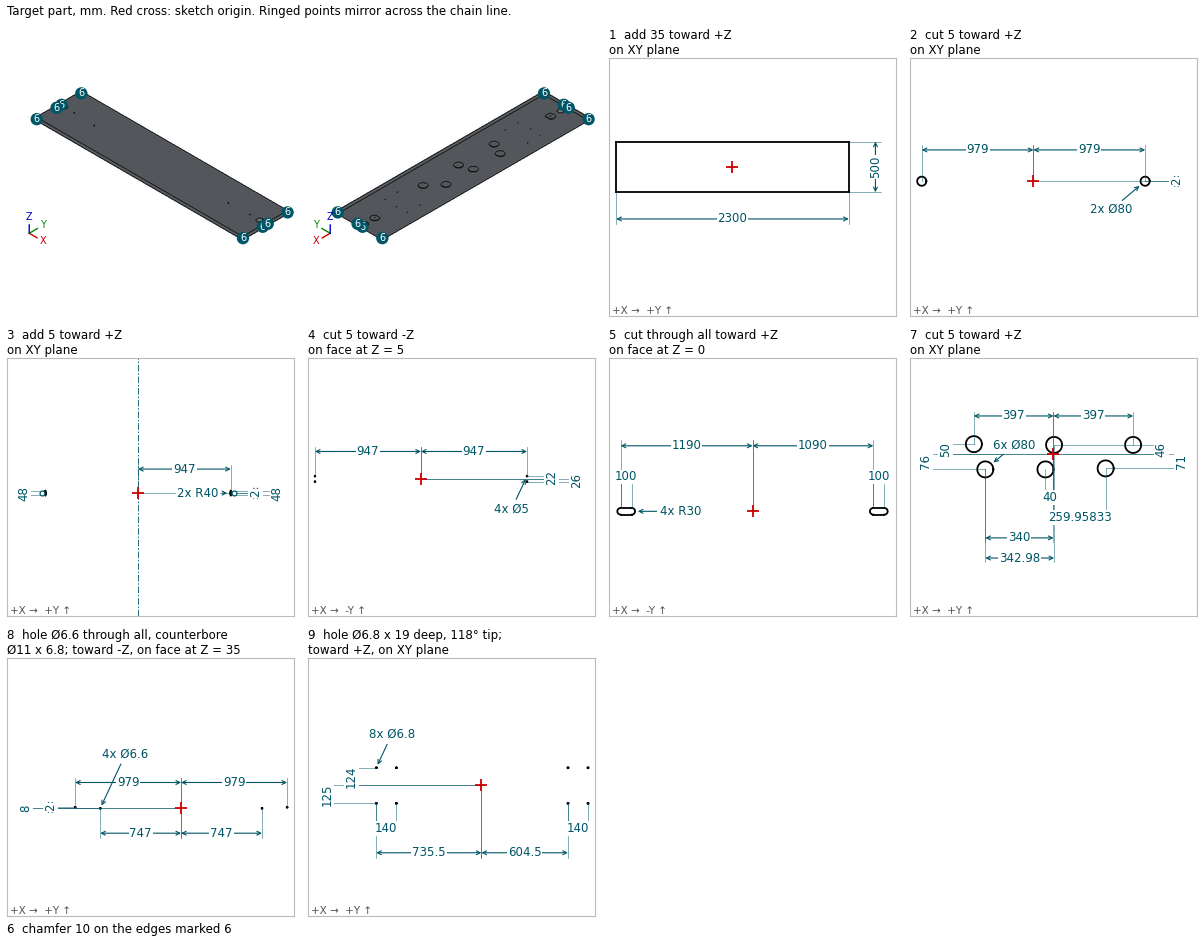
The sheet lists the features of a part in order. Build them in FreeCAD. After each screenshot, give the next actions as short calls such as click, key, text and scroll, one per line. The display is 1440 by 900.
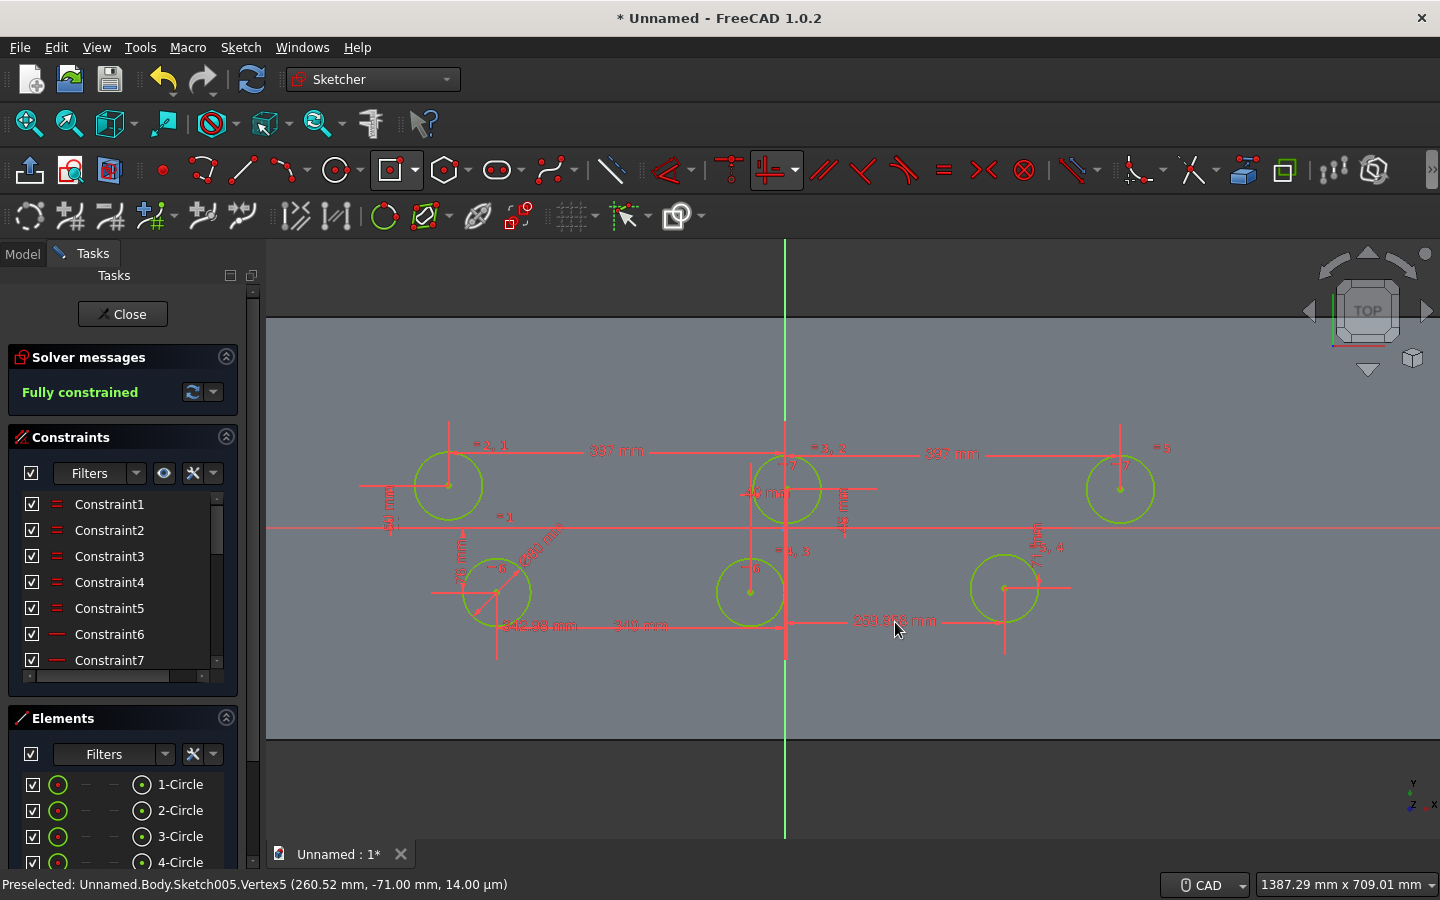
click(123, 314)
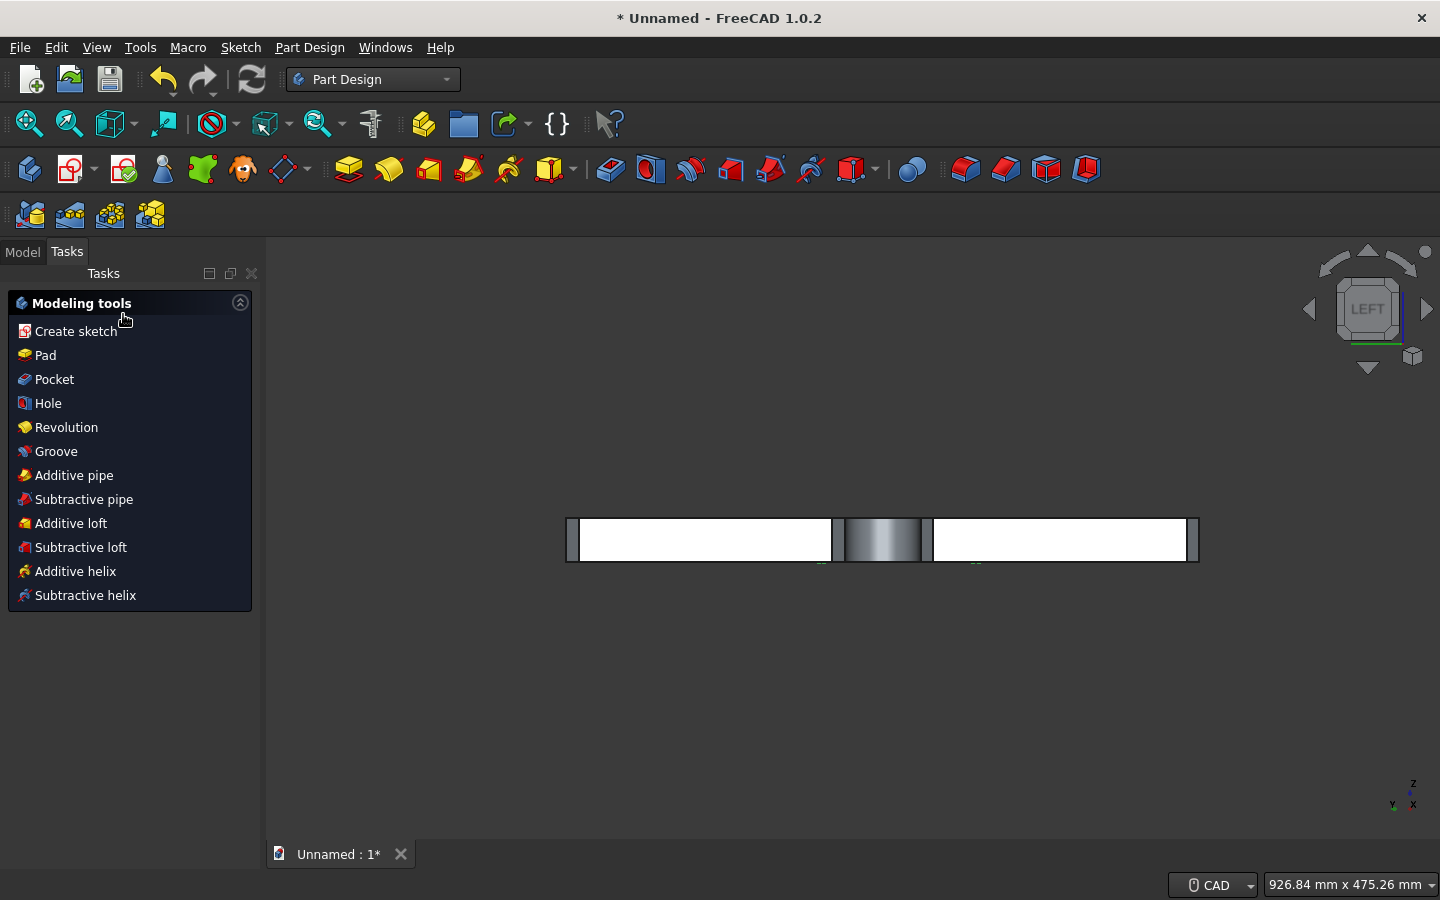
click(612, 170)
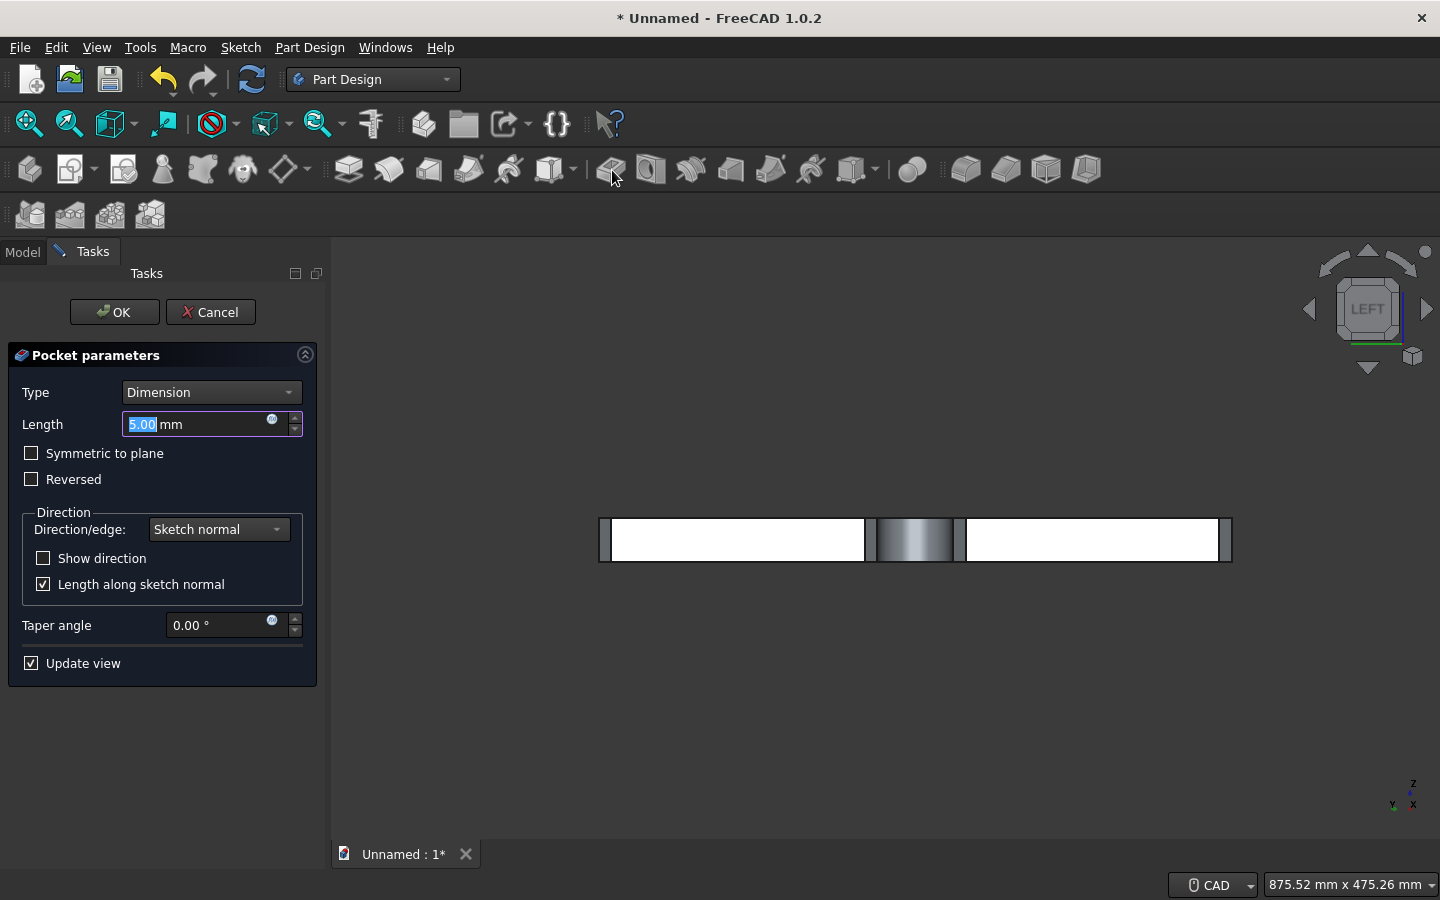
text(5)
key(Tab)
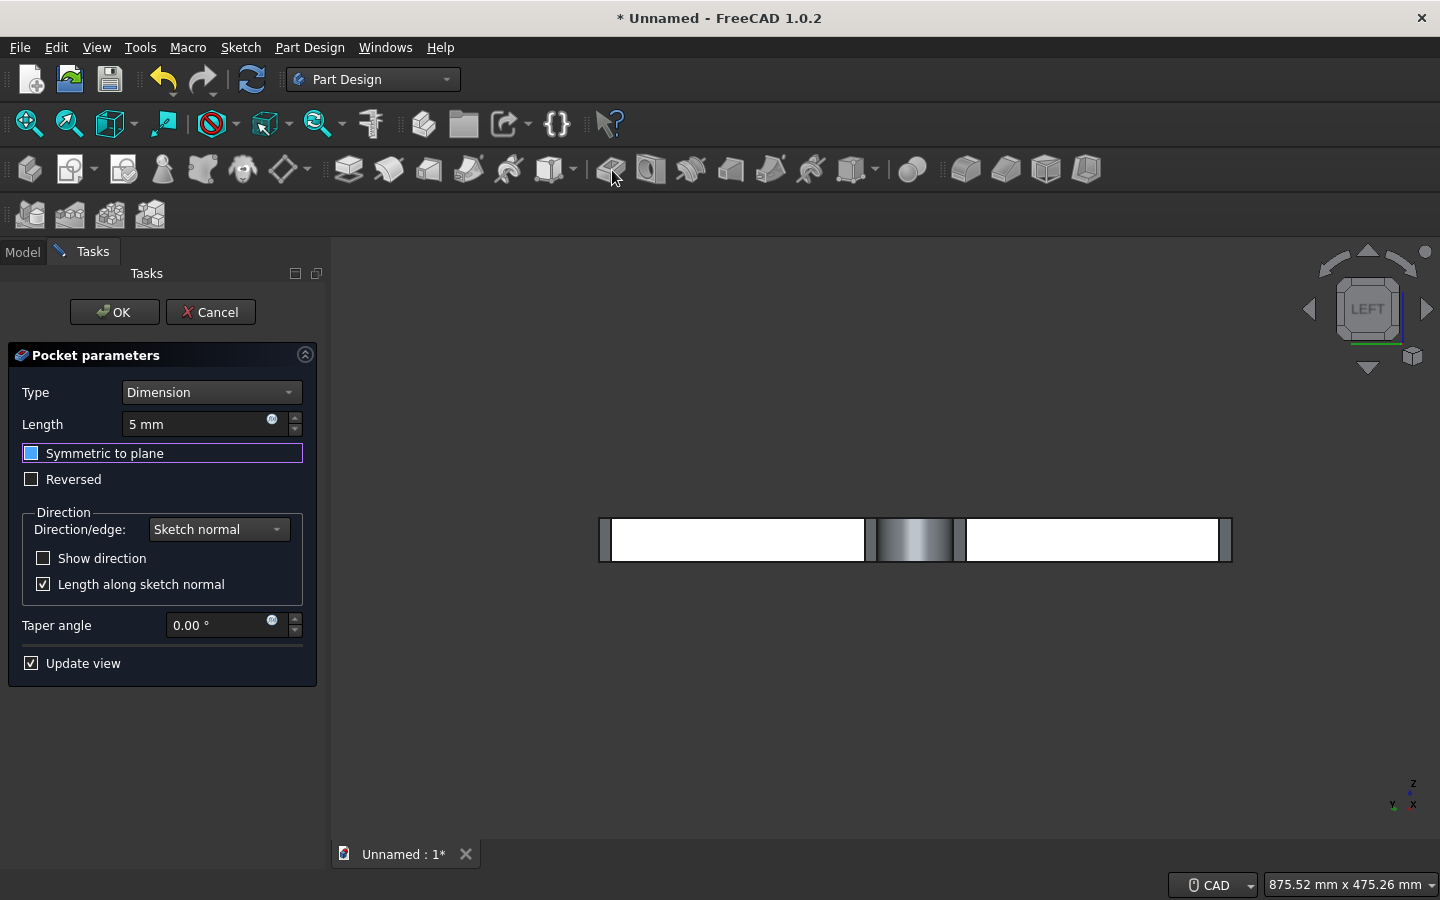
click(30, 479)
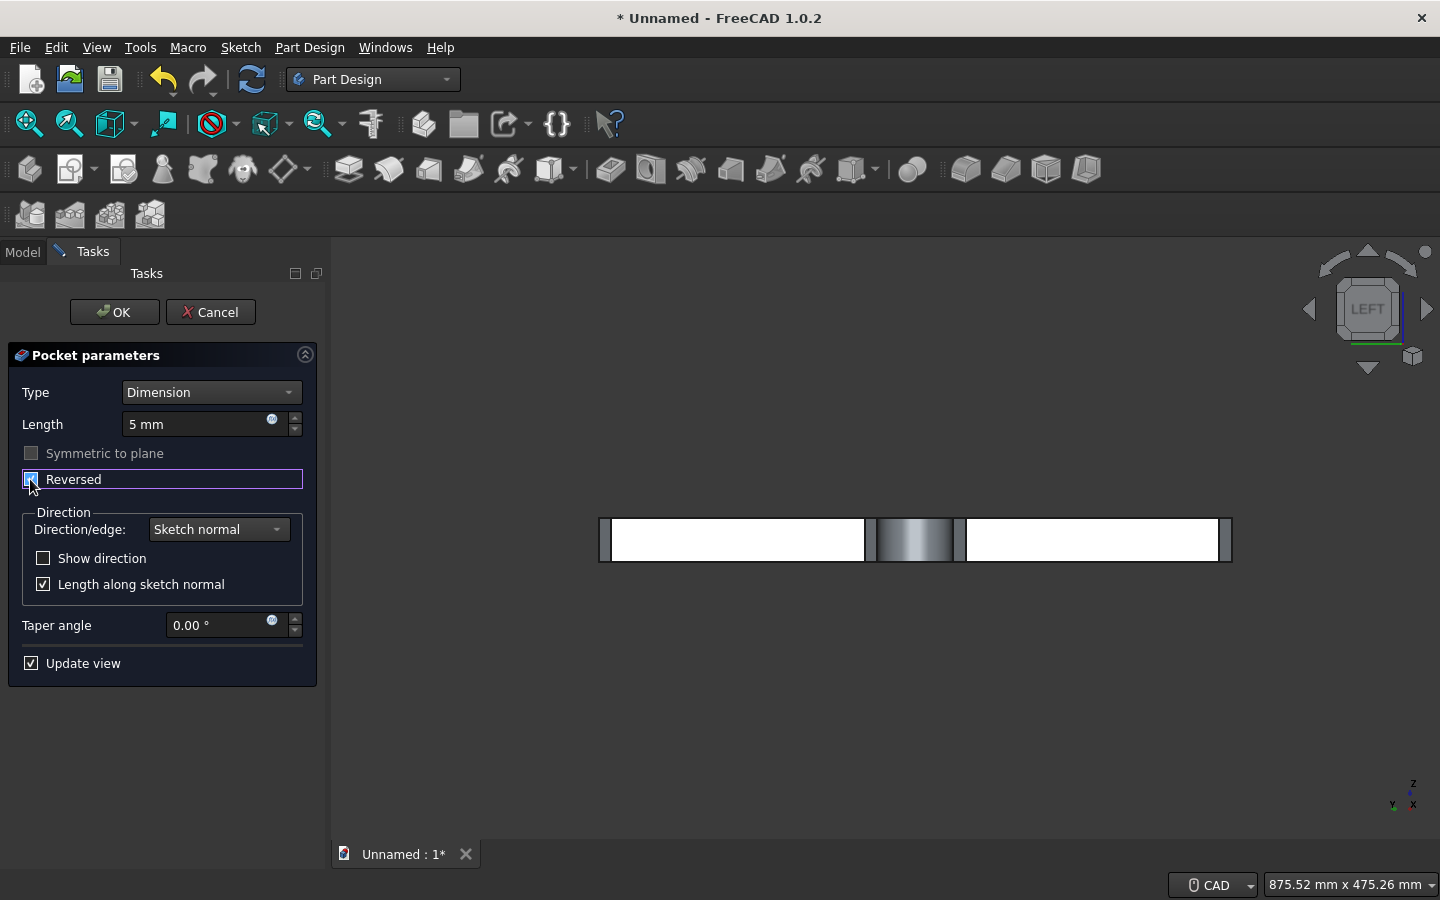
click(115, 312)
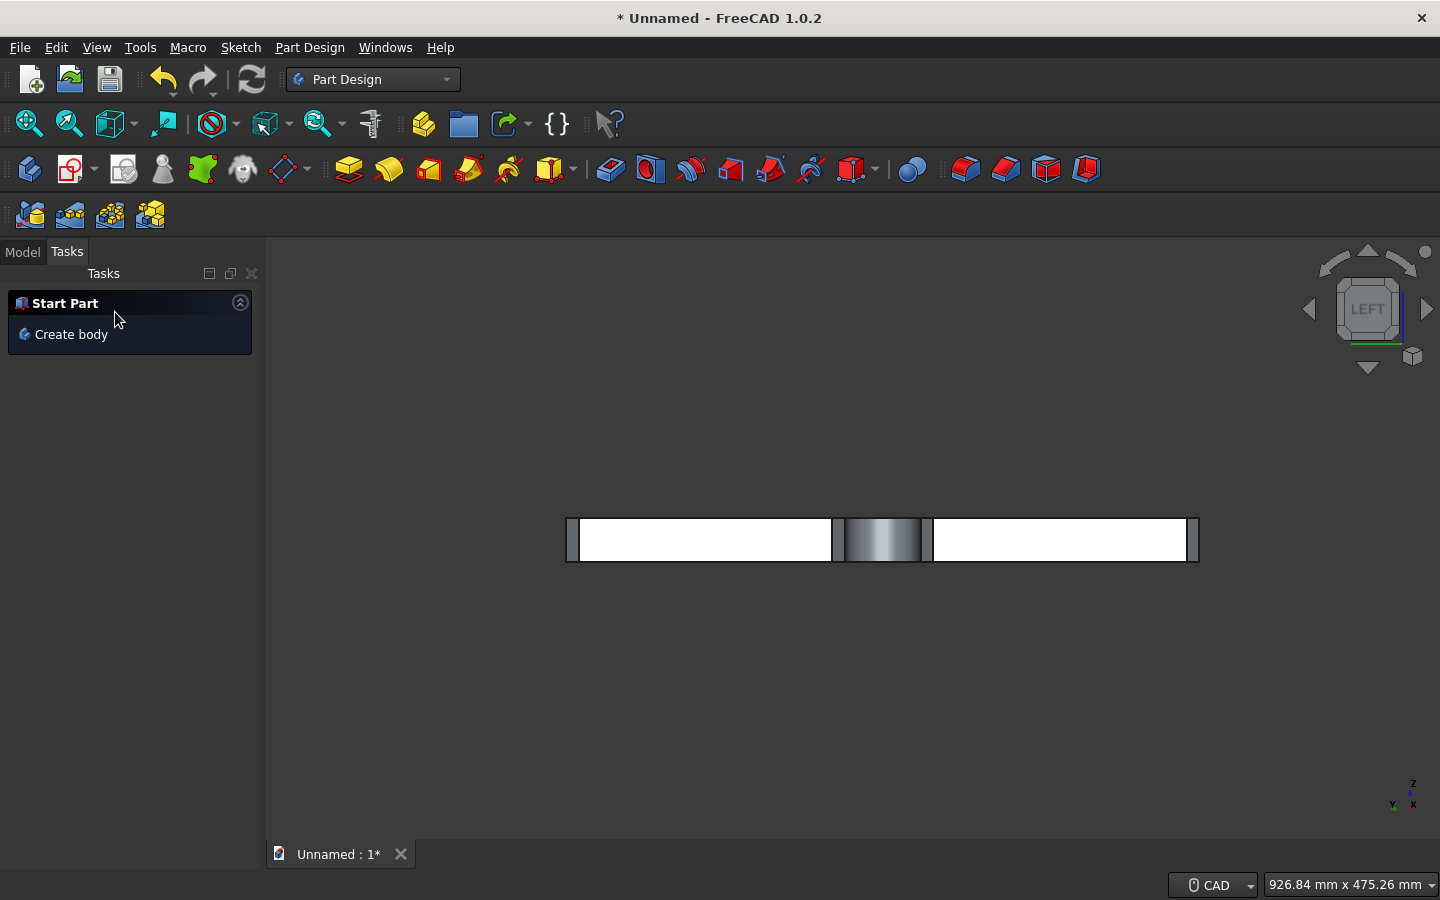
key(0)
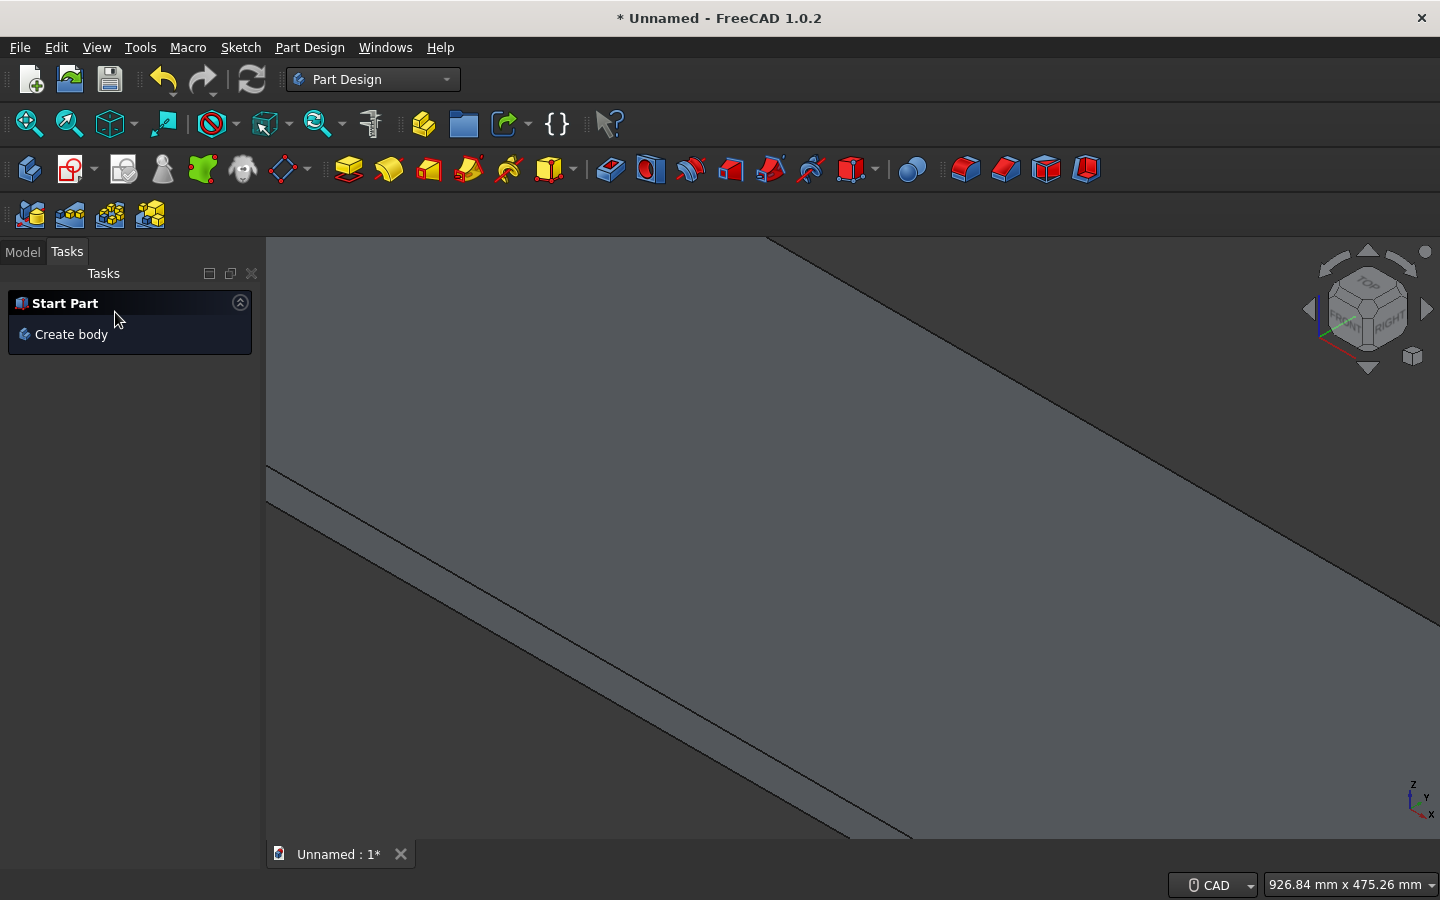
click(30, 124)